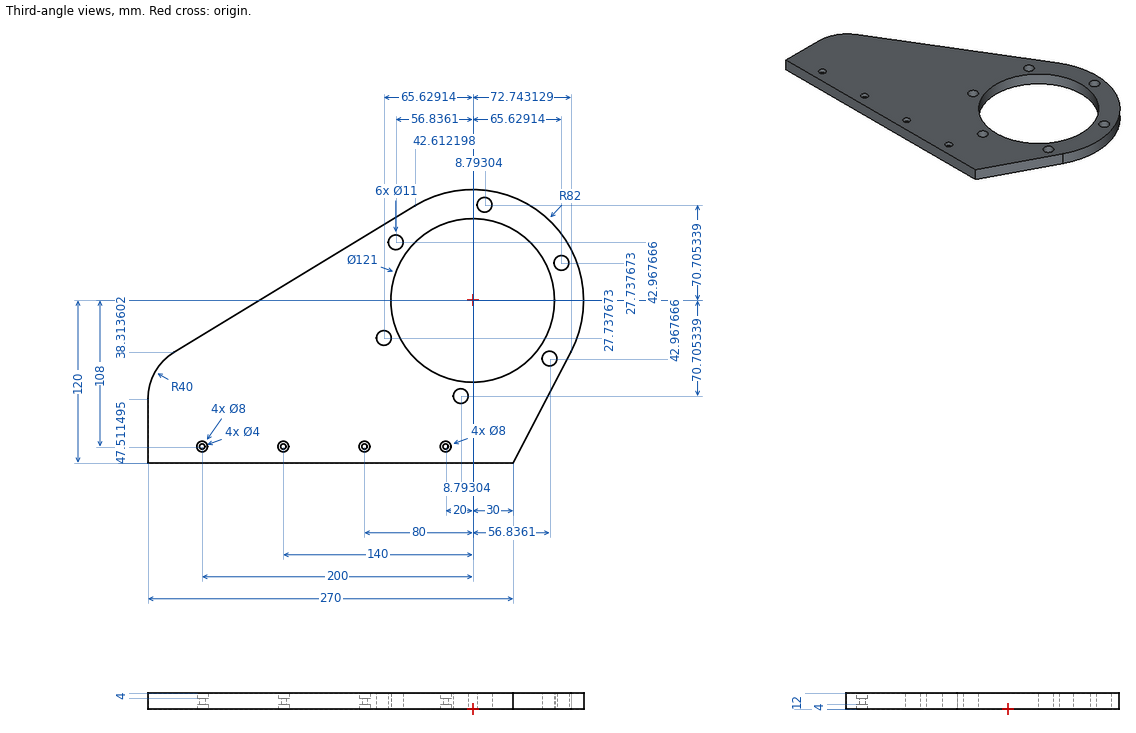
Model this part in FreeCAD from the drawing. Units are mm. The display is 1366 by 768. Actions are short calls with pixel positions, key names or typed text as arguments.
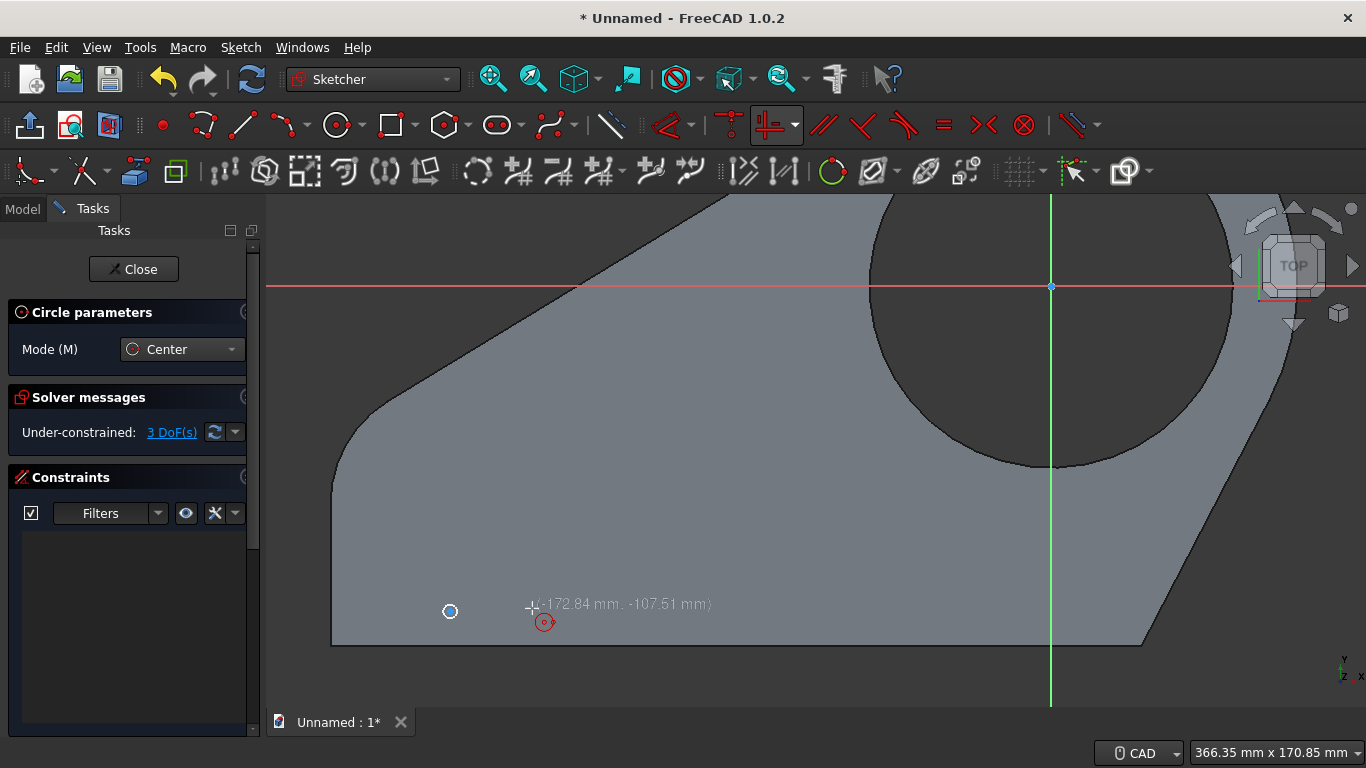
click(631, 610)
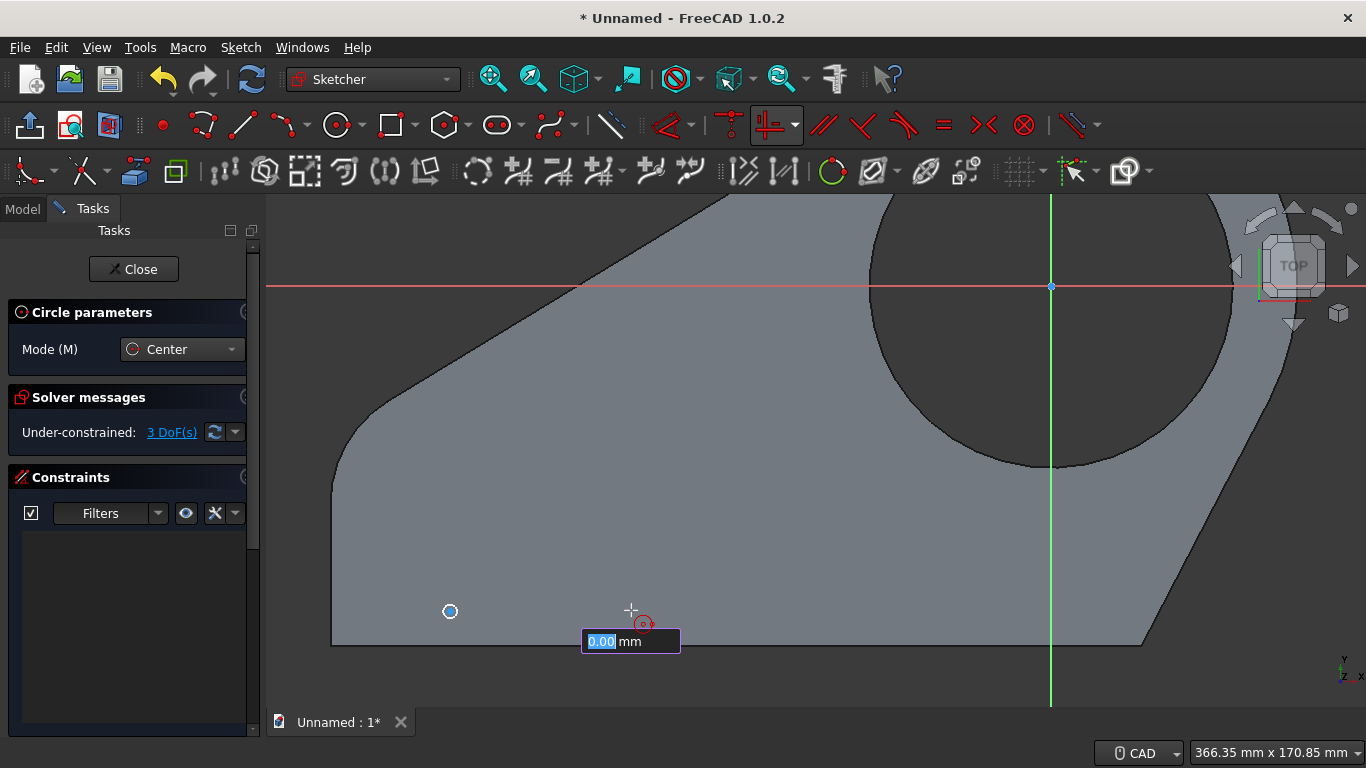
scroll(635, 606, up, 5)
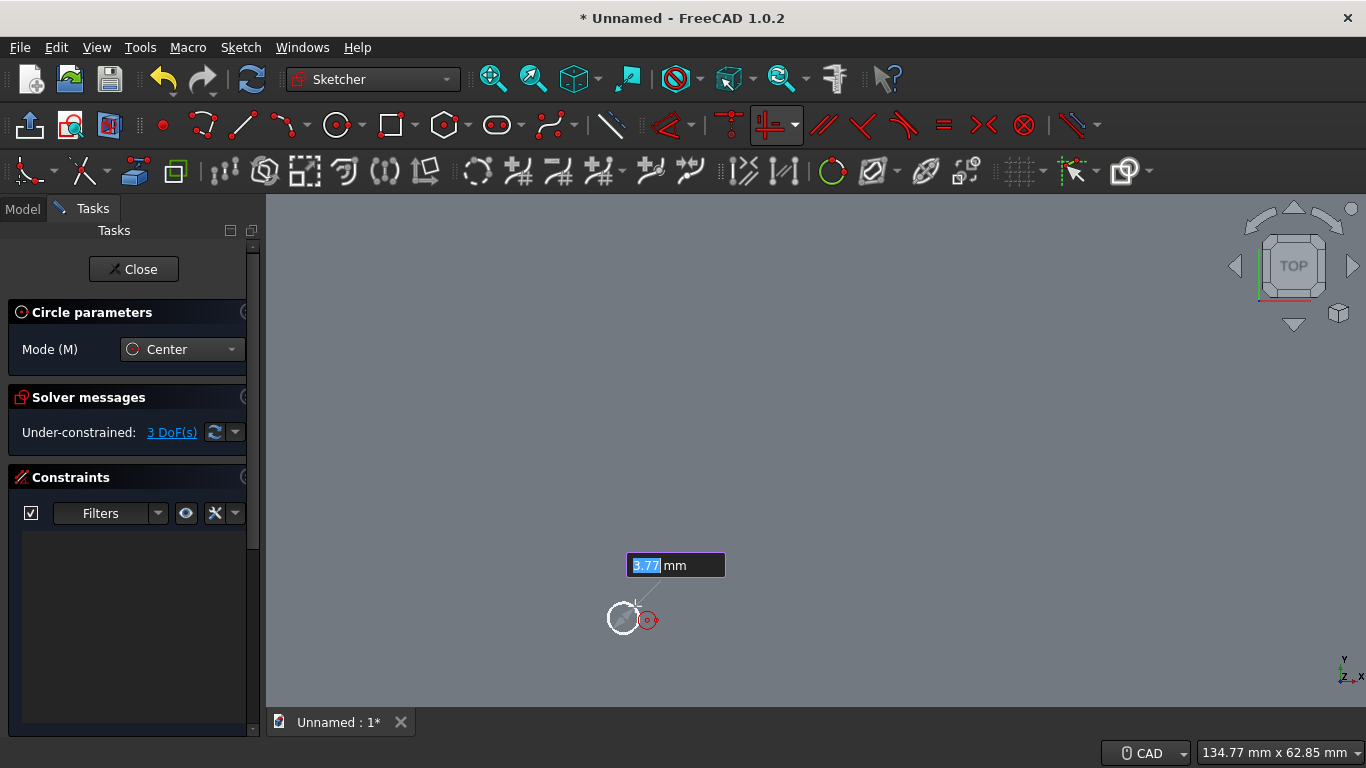
click(635, 605)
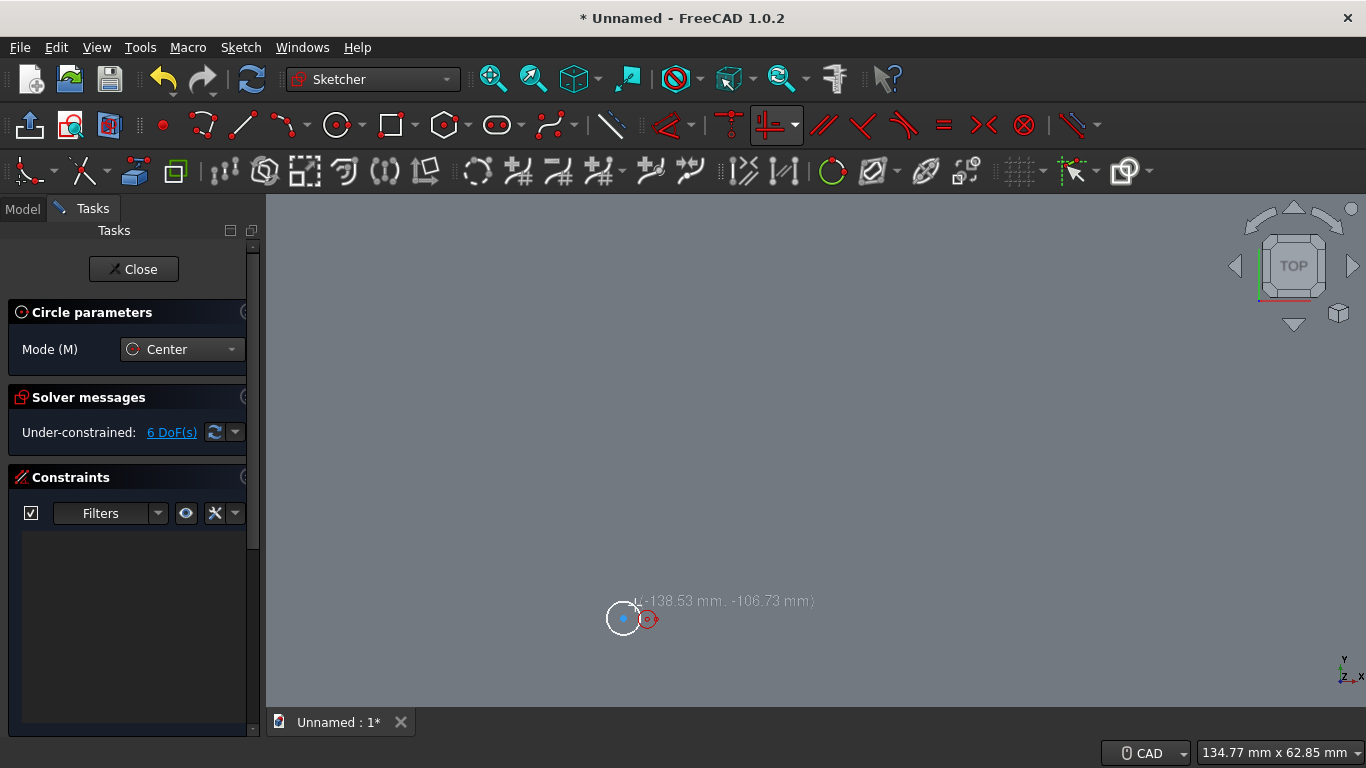
scroll(1113, 616, up, 2)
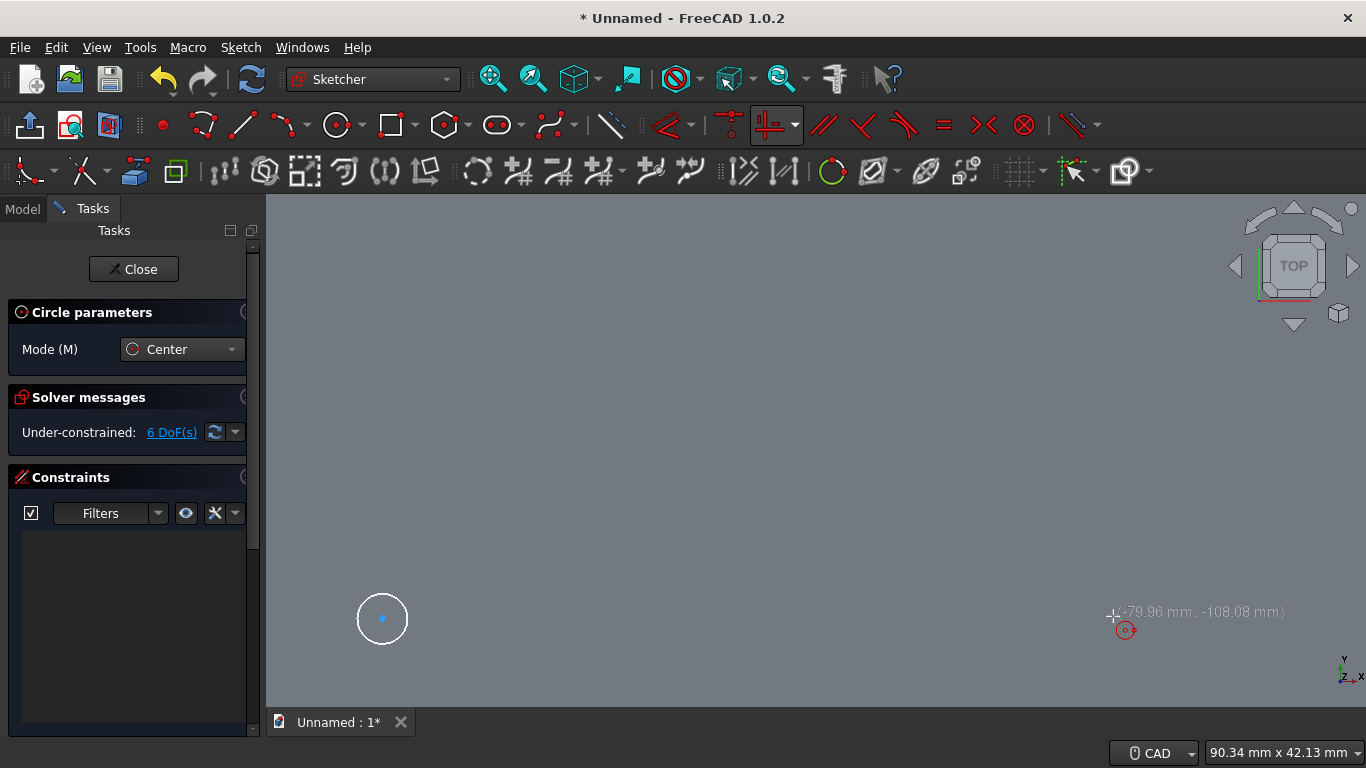
scroll(712, 608, down, 7)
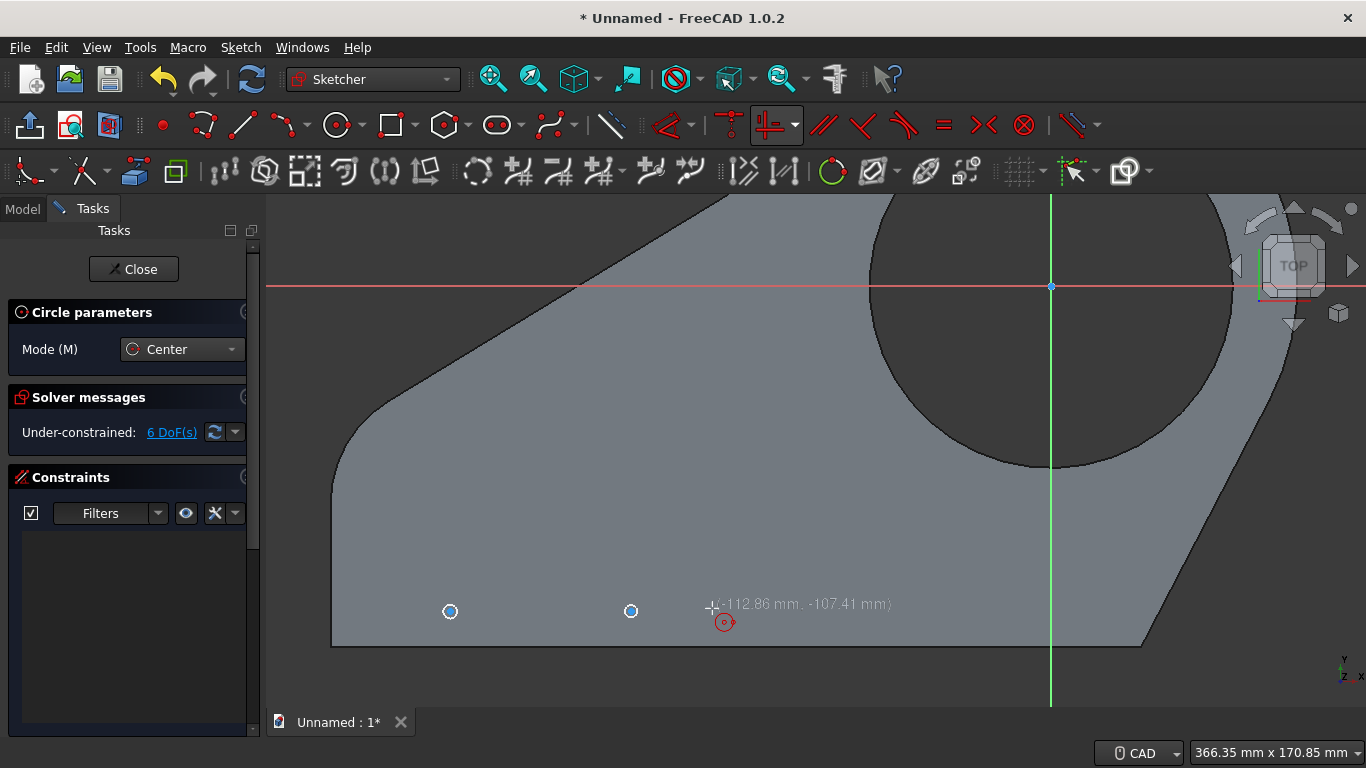
click(811, 611)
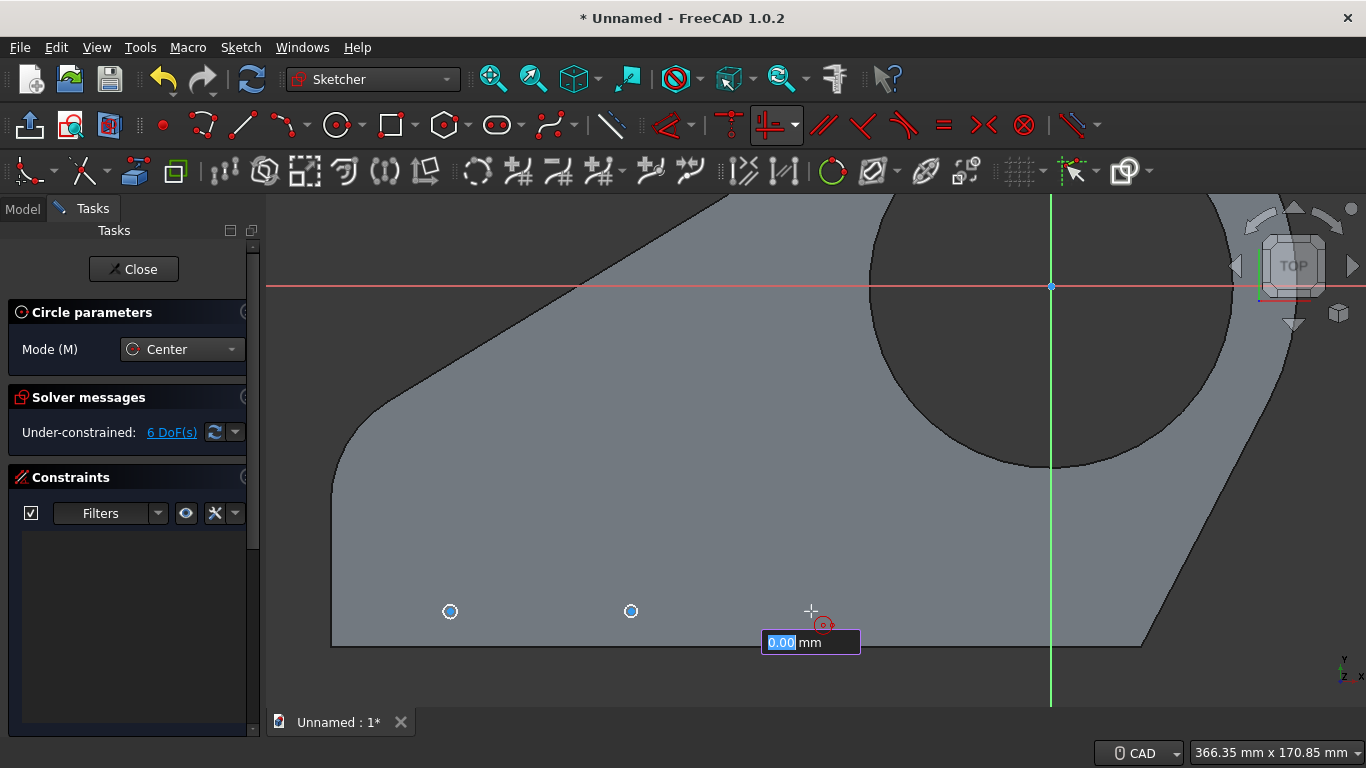
scroll(815, 606, up, 5)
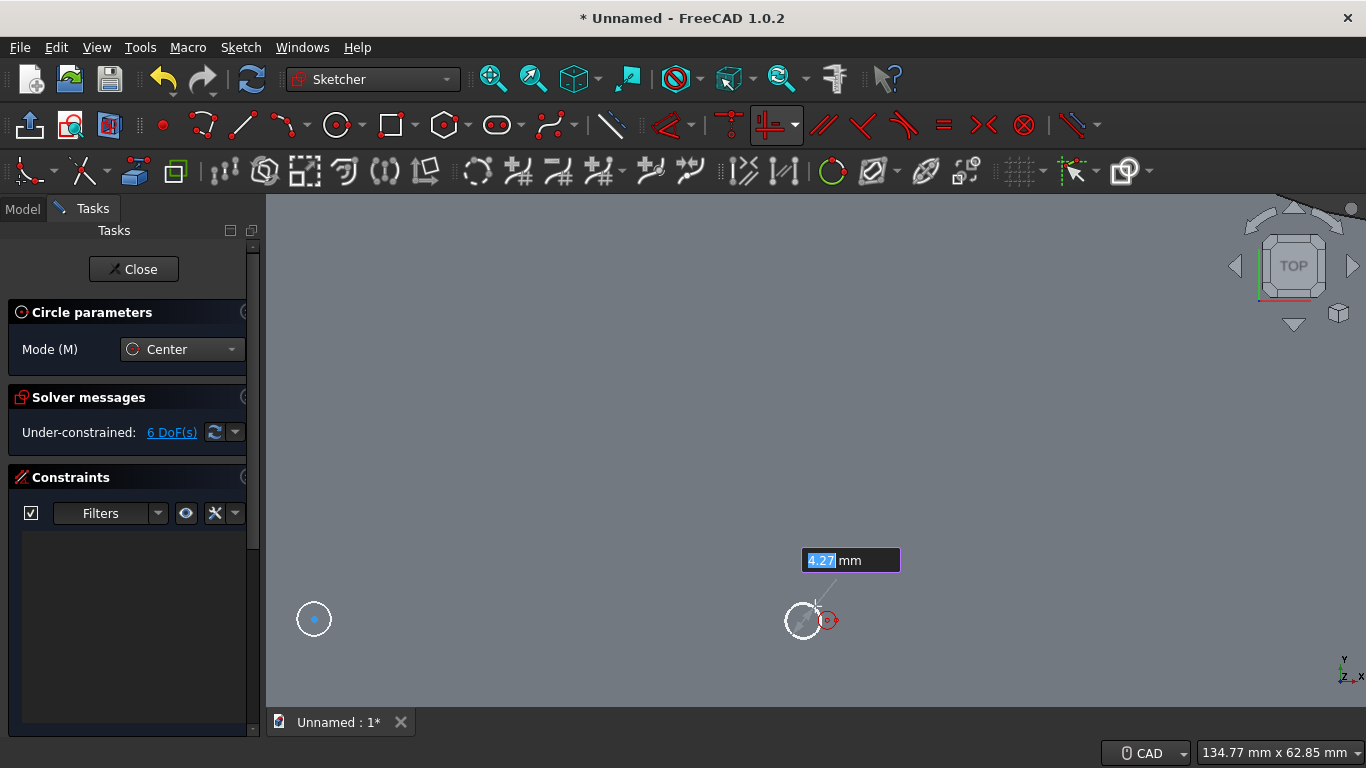
click(815, 606)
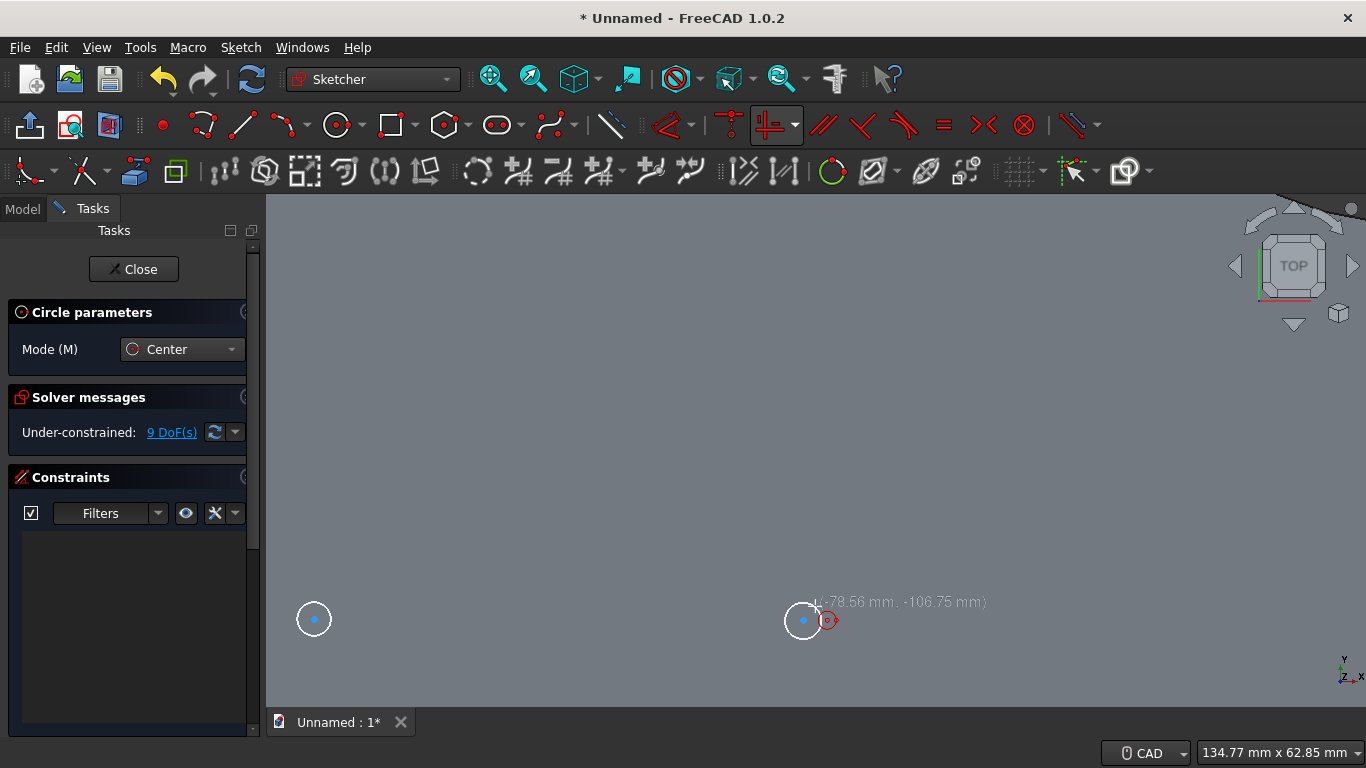
scroll(815, 605, down, 5)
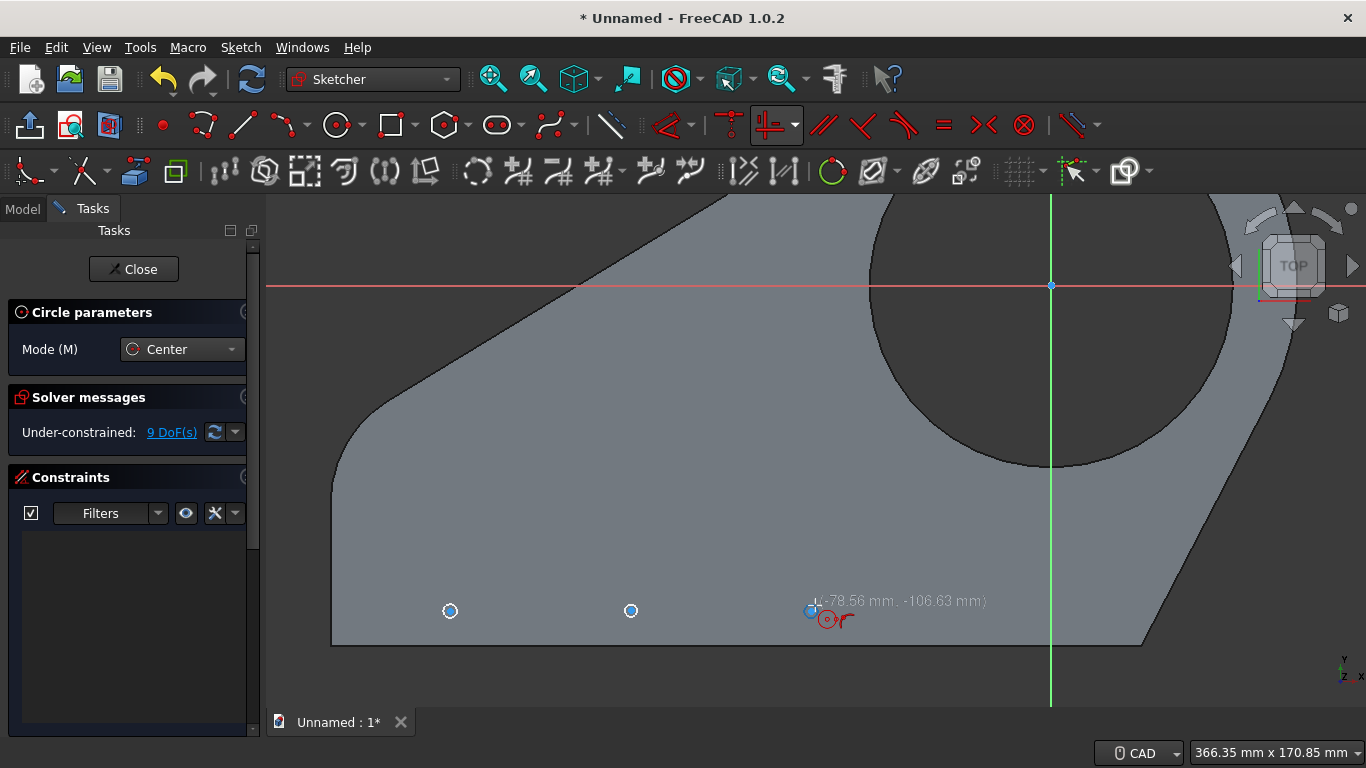
scroll(991, 610, up, 7)